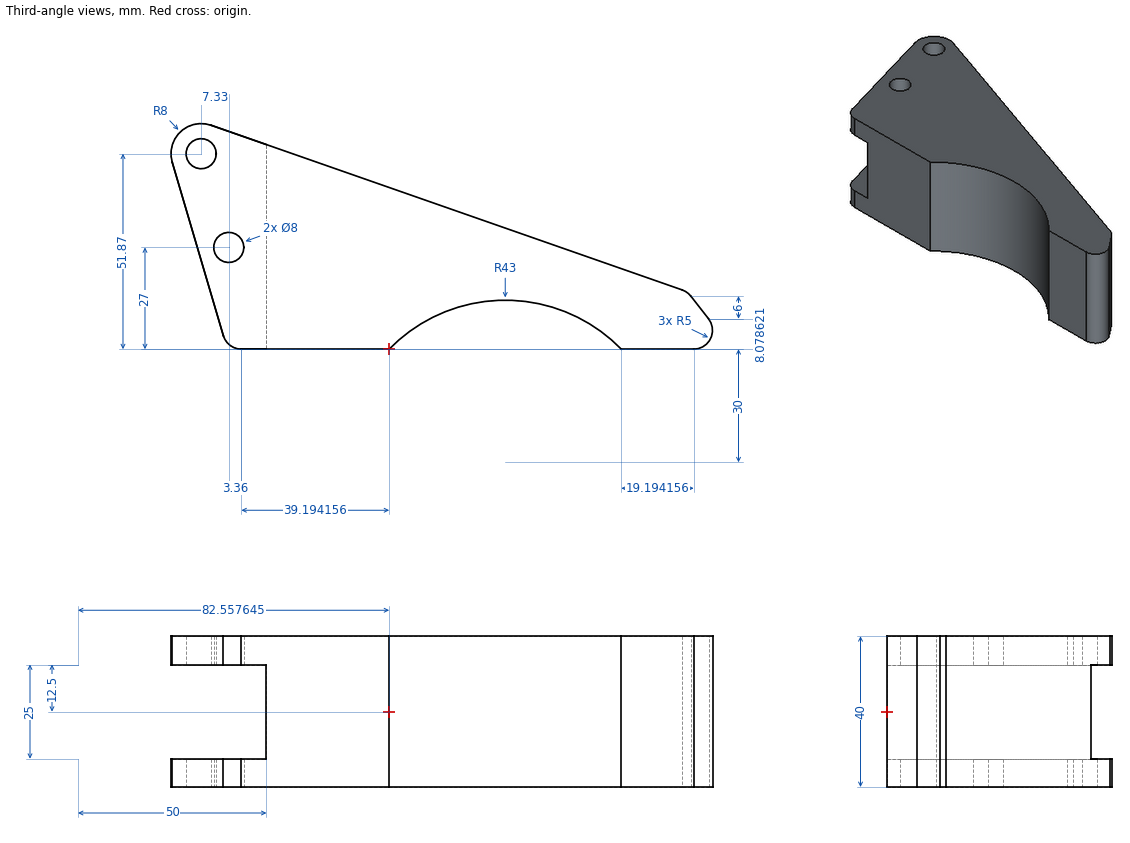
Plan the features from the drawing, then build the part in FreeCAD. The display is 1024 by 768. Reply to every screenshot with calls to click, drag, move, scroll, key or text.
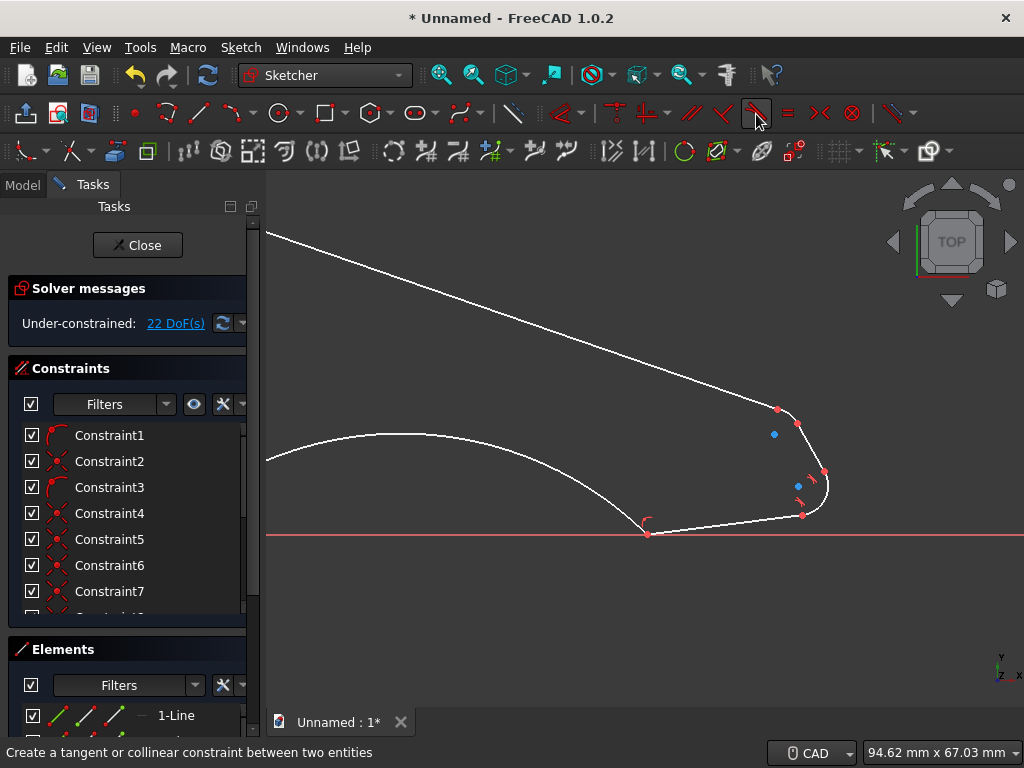
click(816, 457)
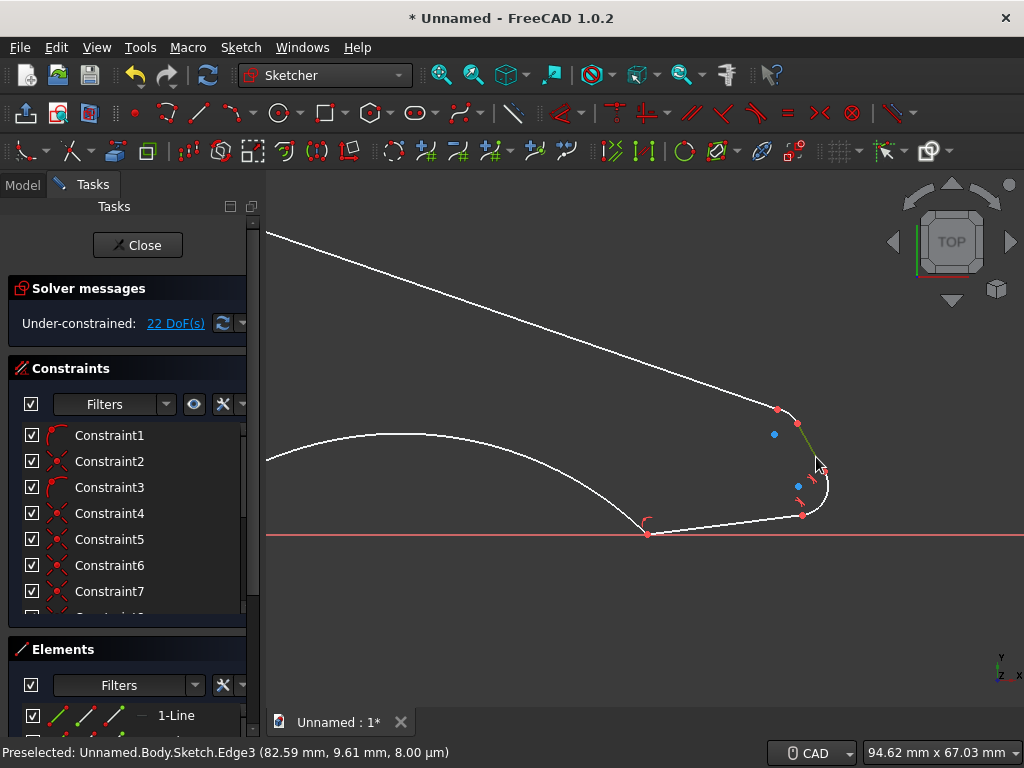
click(789, 414)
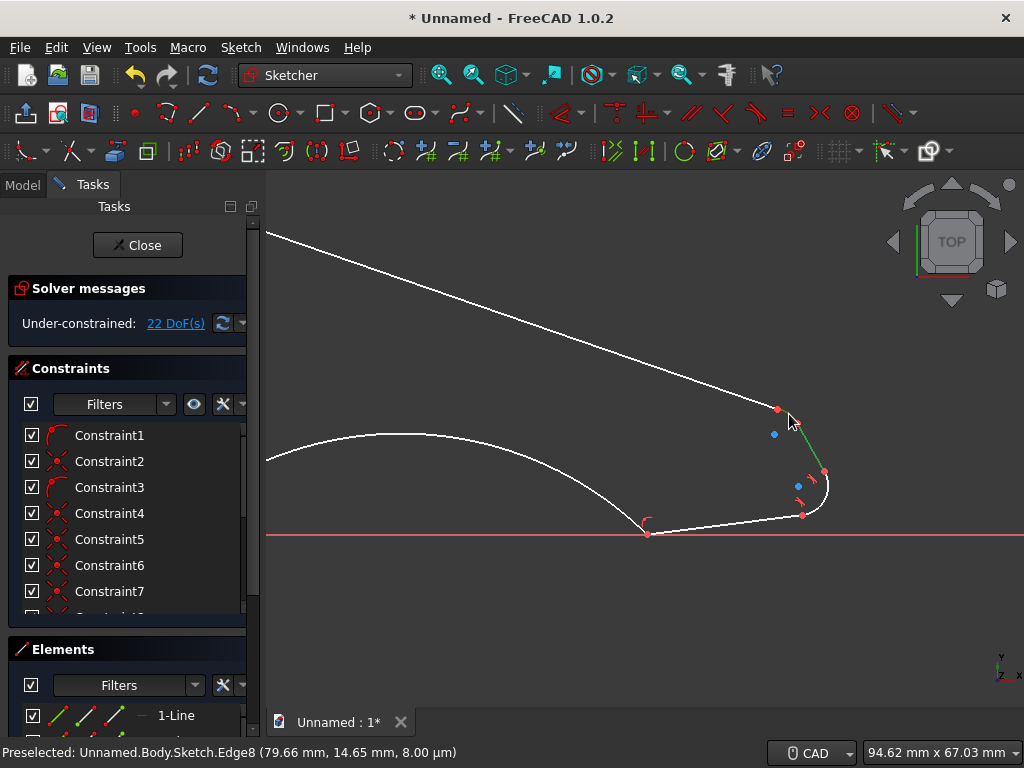
key(t)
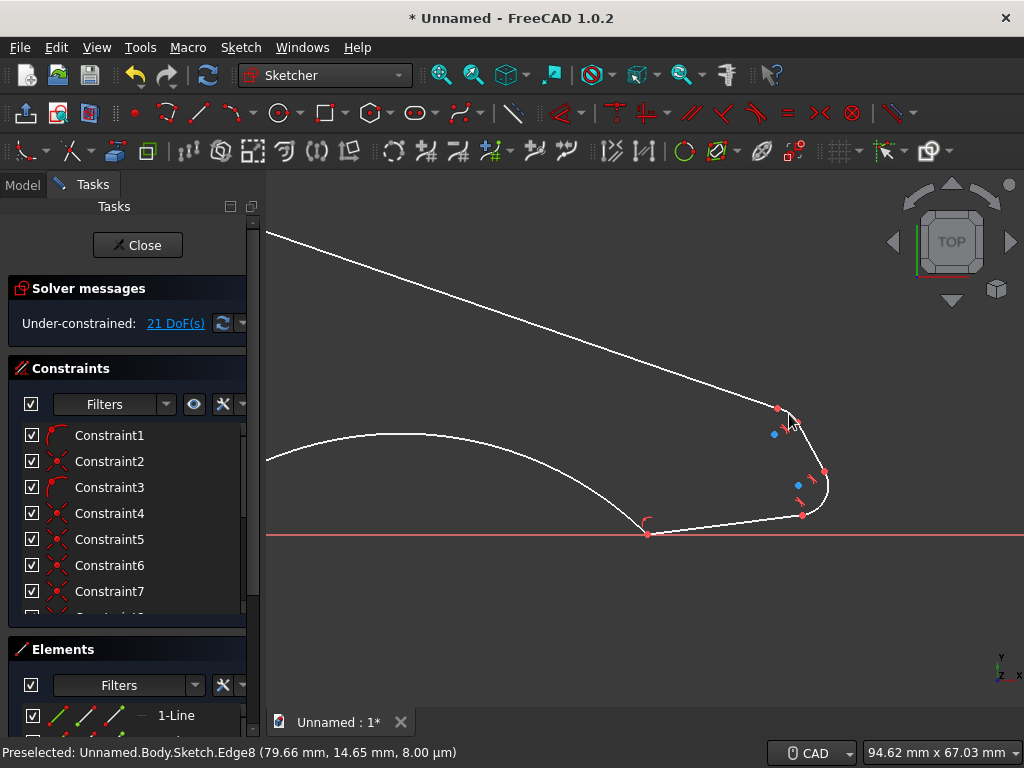
click(477, 305)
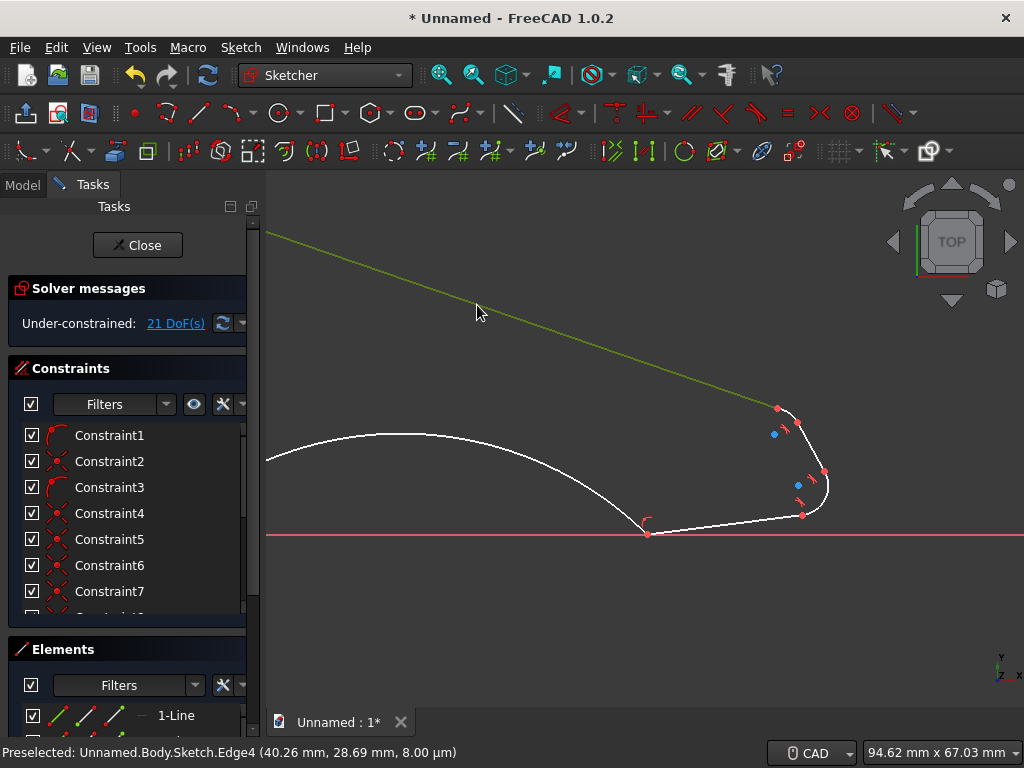
click(789, 413)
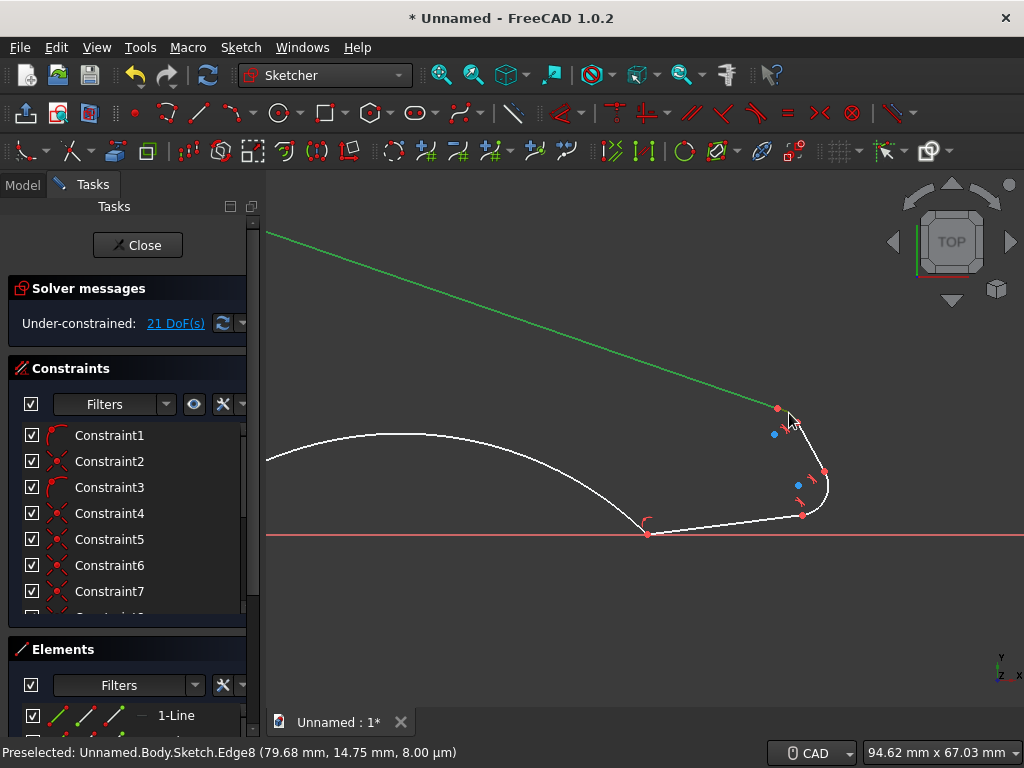
click(756, 114)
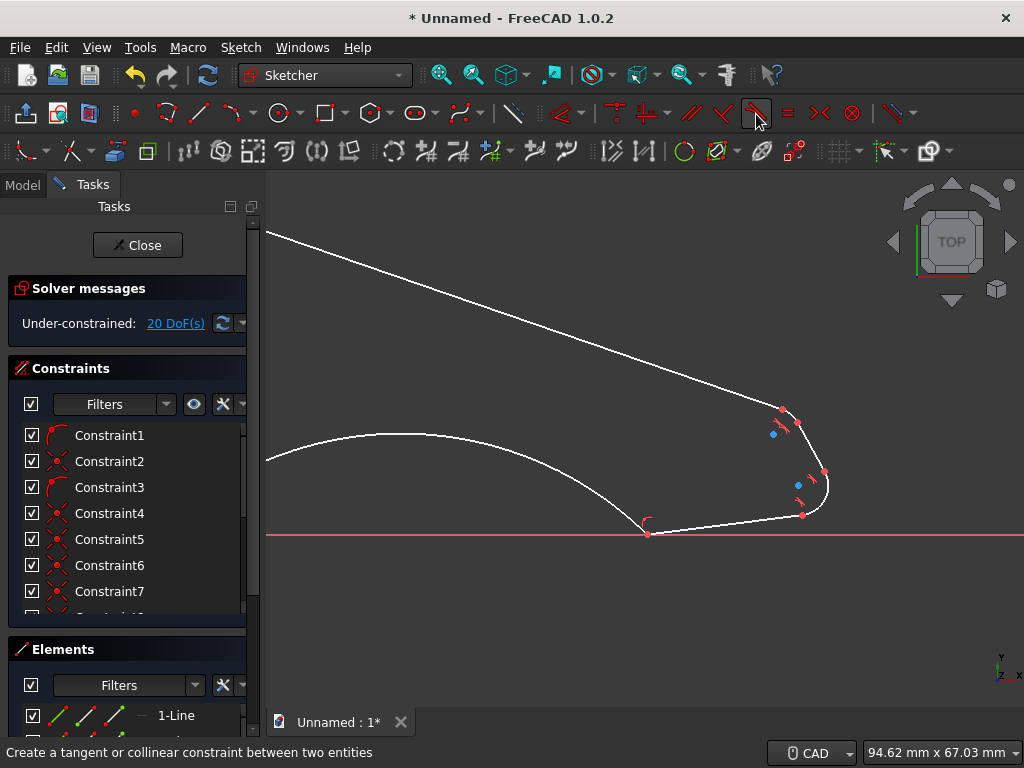
click(481, 306)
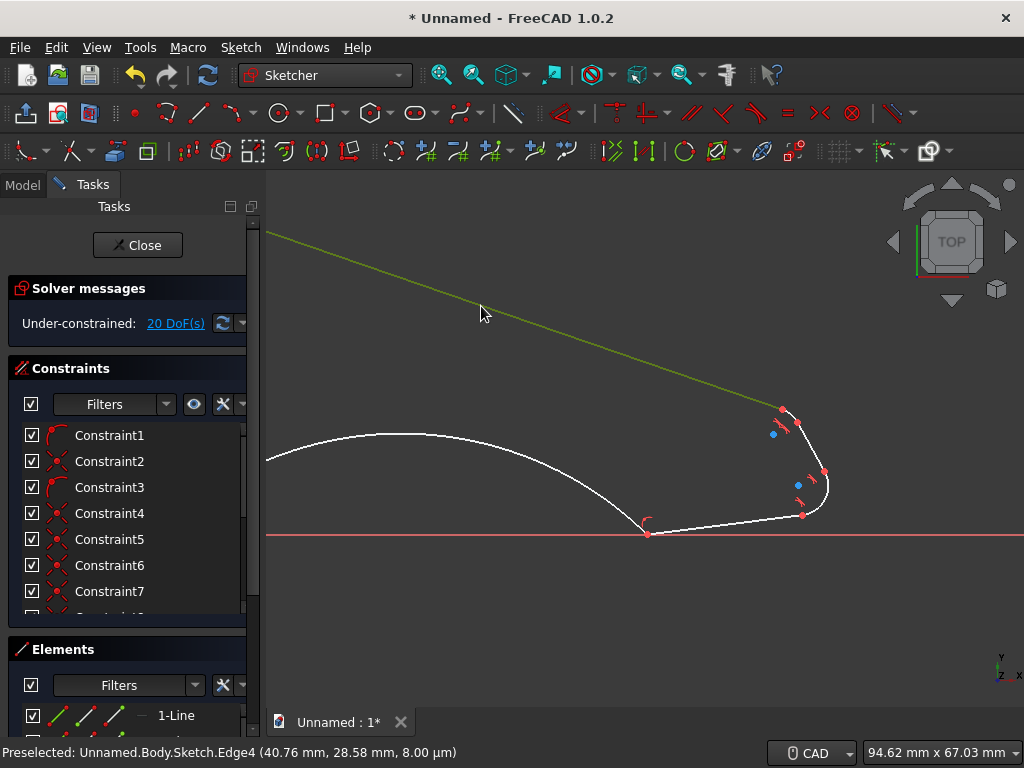
scroll(757, 521, down, 5)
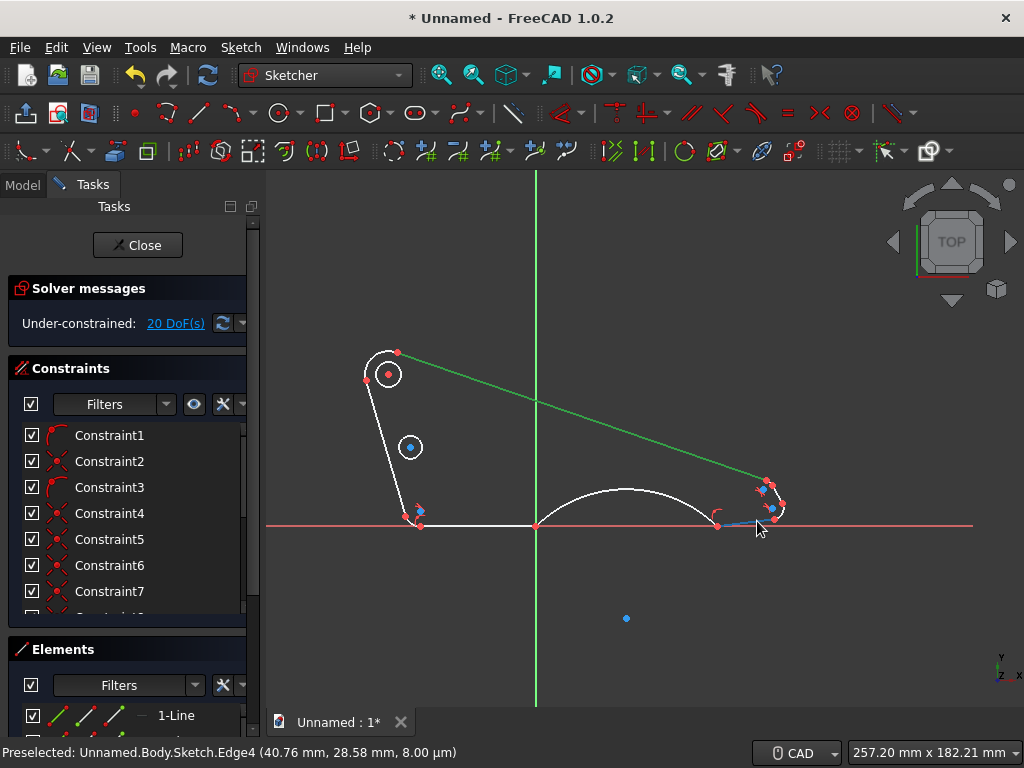
scroll(382, 352, up, 2)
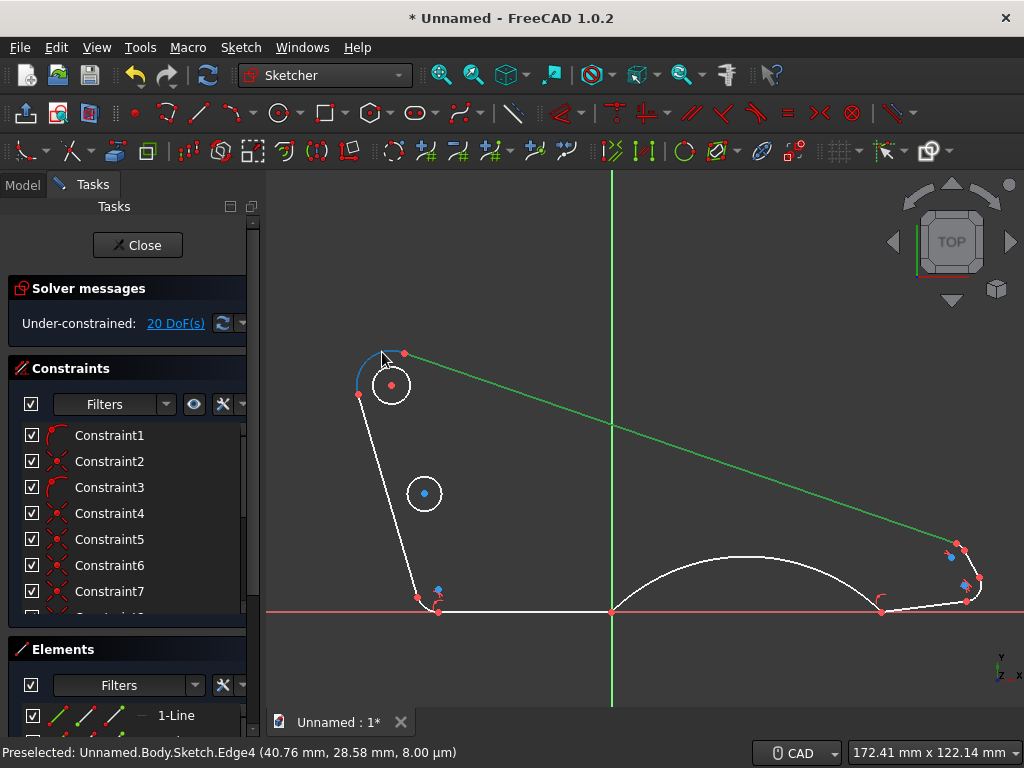
click(382, 352)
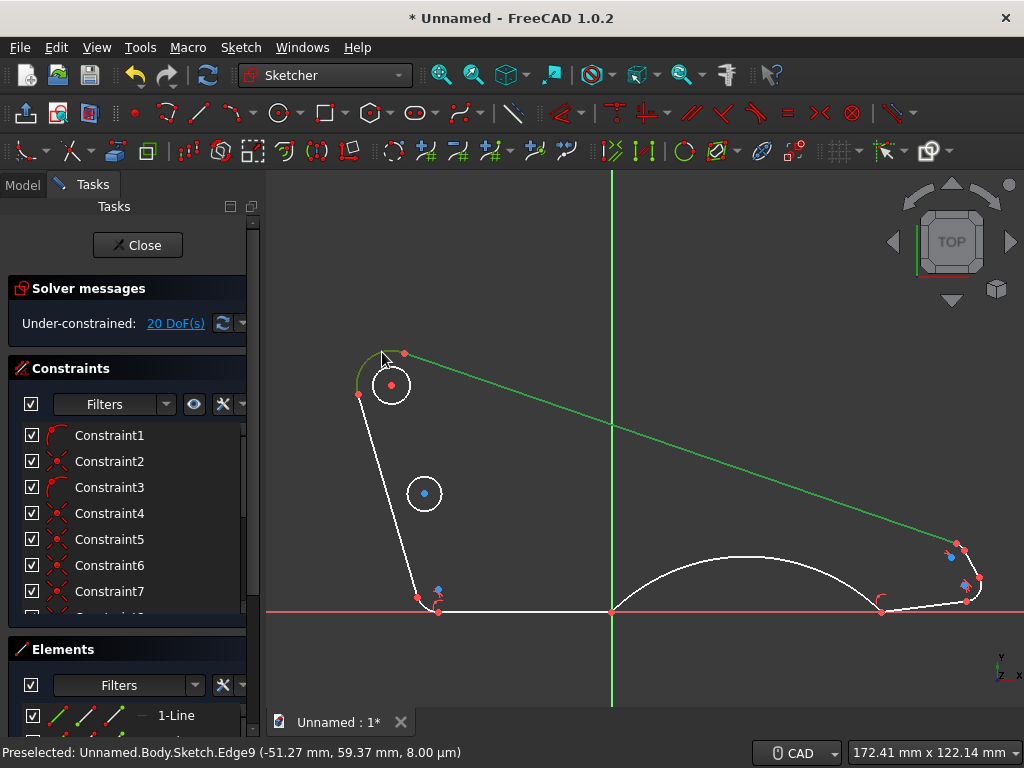
click(756, 114)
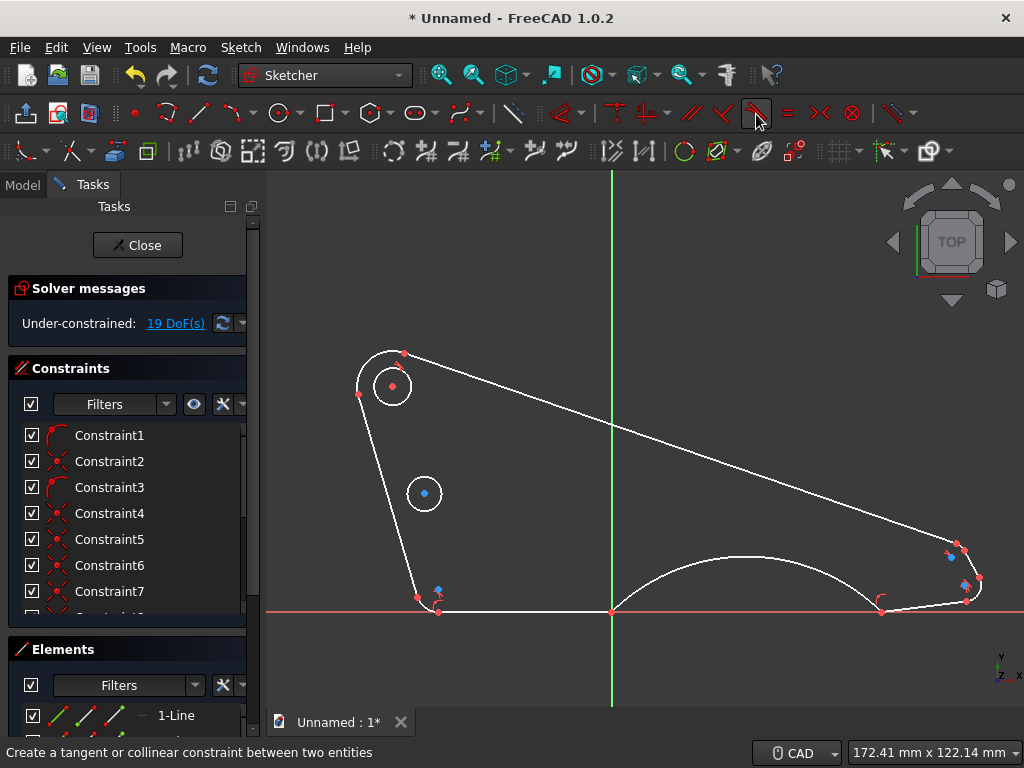
click(376, 456)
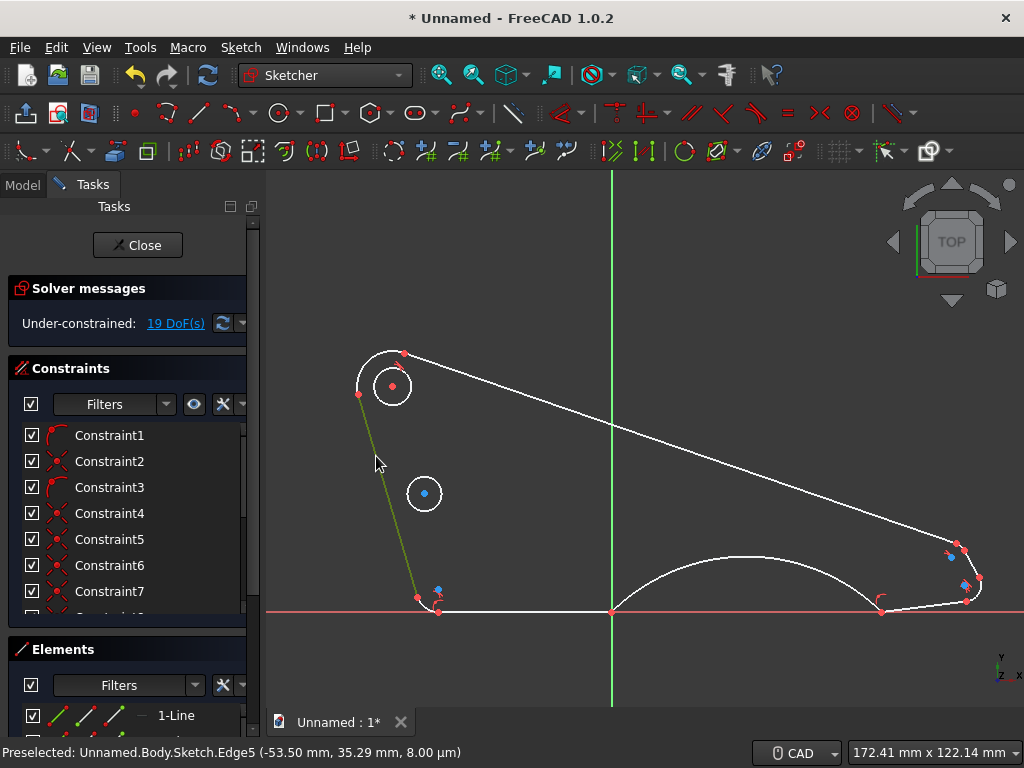
click(382, 353)